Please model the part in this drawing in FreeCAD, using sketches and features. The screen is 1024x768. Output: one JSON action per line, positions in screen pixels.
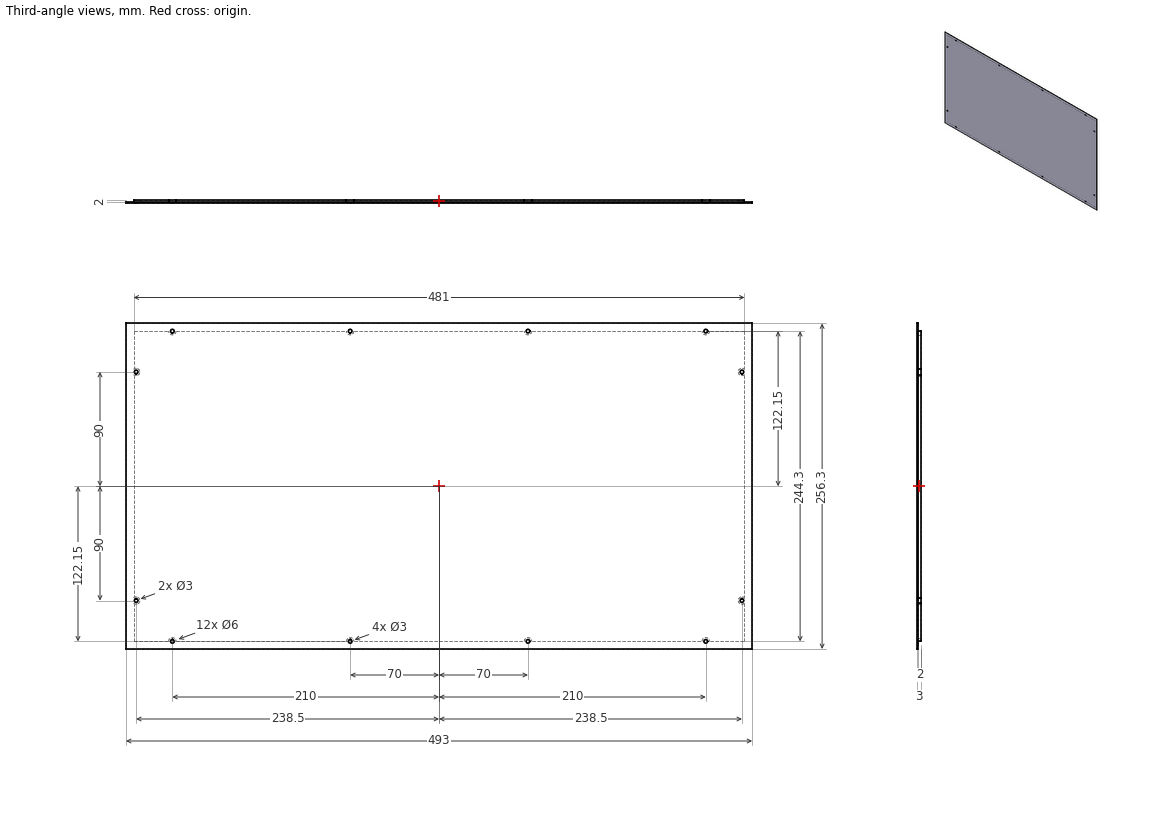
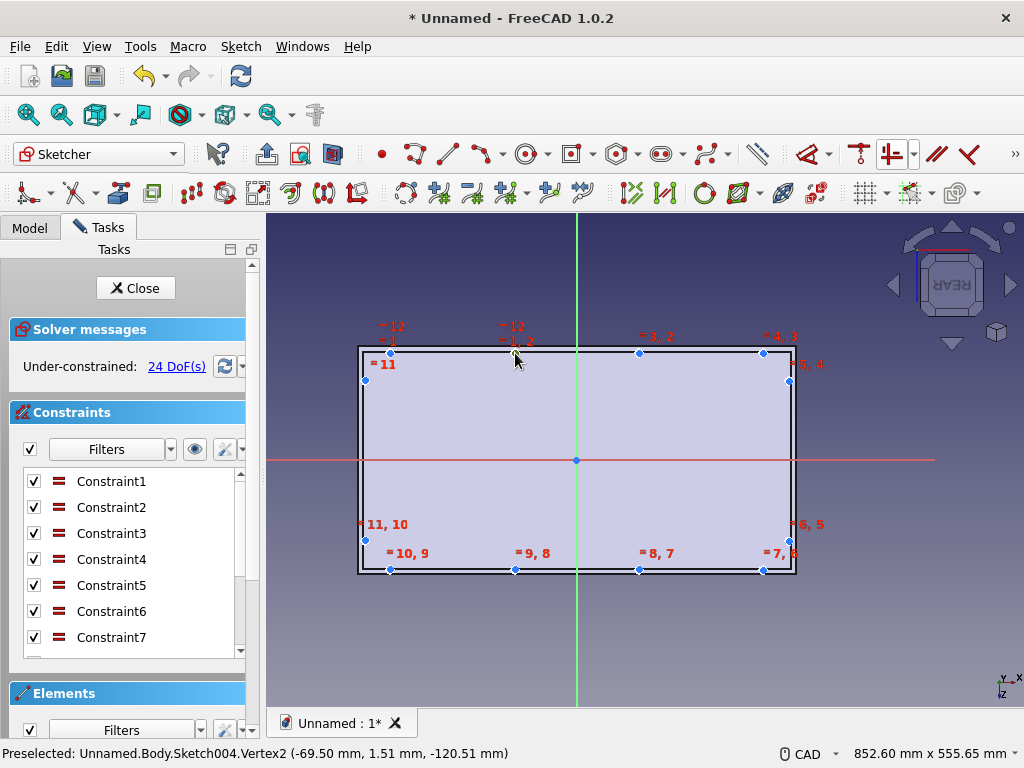
{"action": "left_click", "coordinate": [639, 353]}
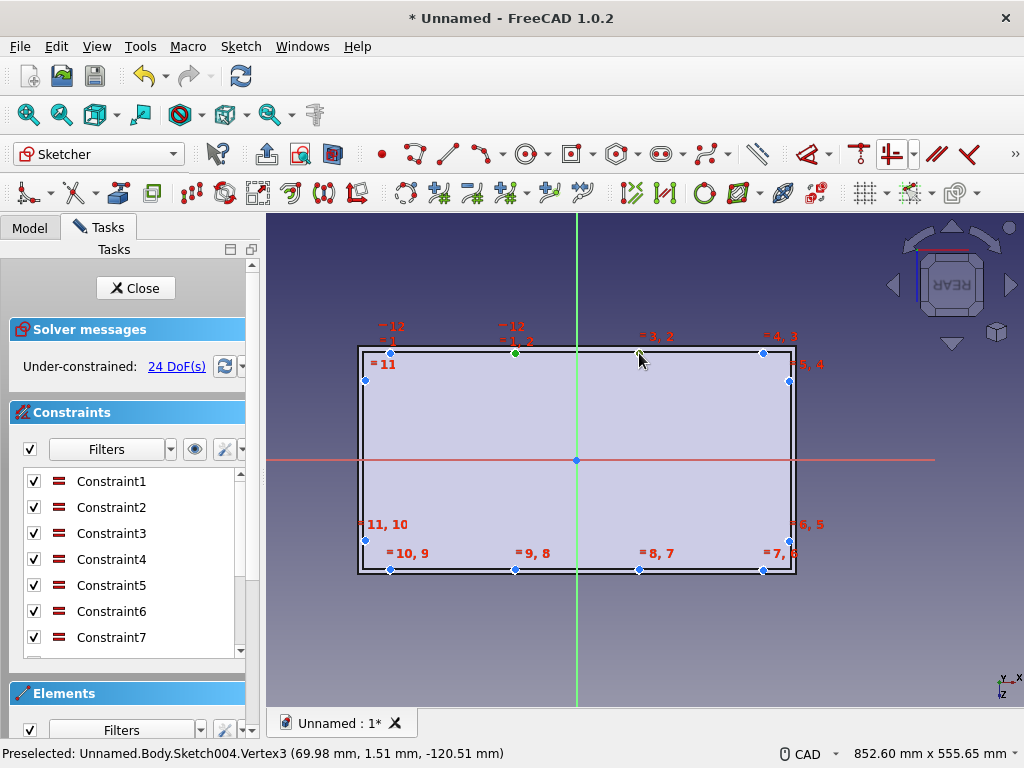
{"action": "left_click", "coordinate": [914, 154]}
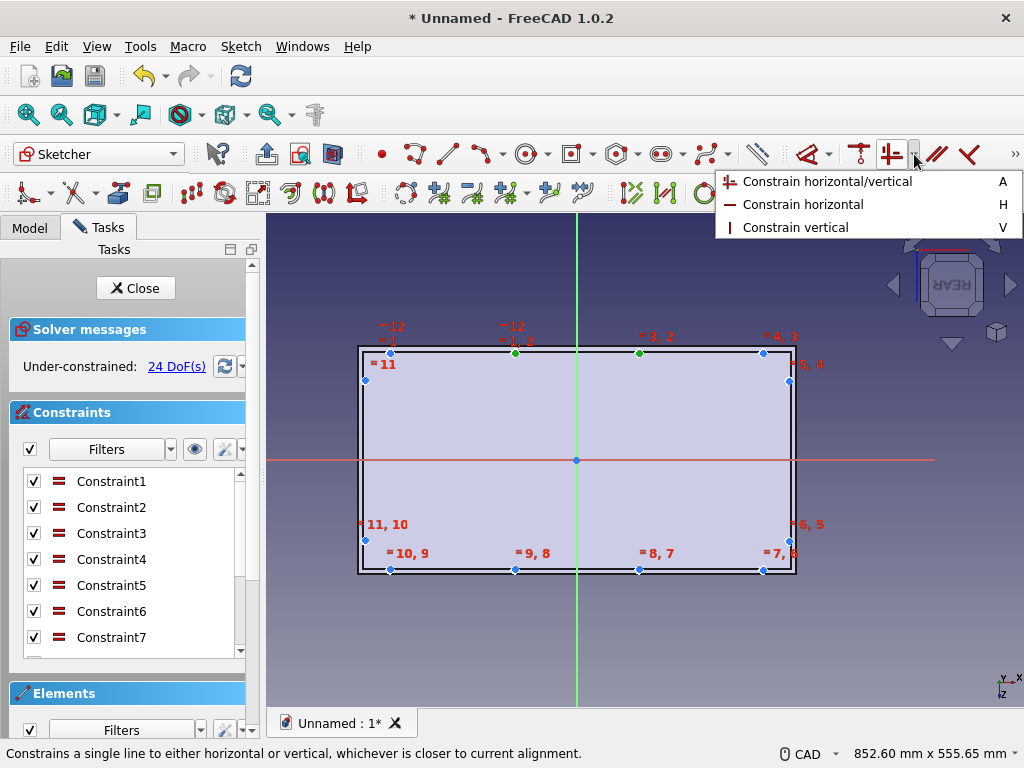
{"action": "left_click", "coordinate": [869, 204]}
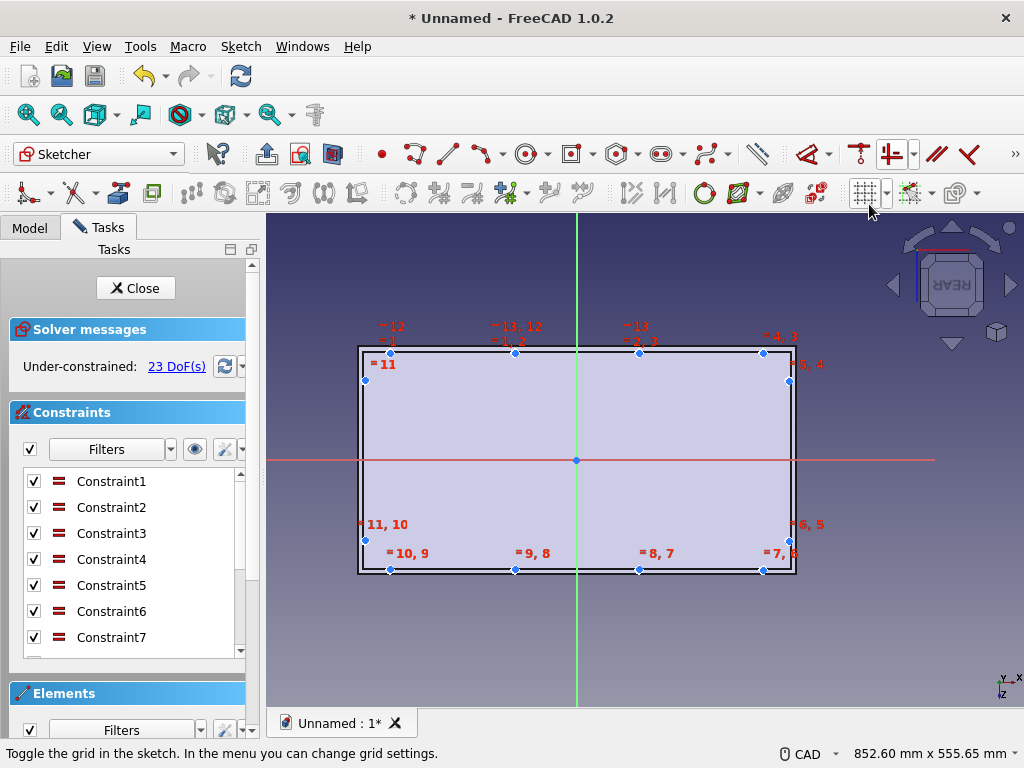
{"action": "left_click", "coordinate": [639, 353]}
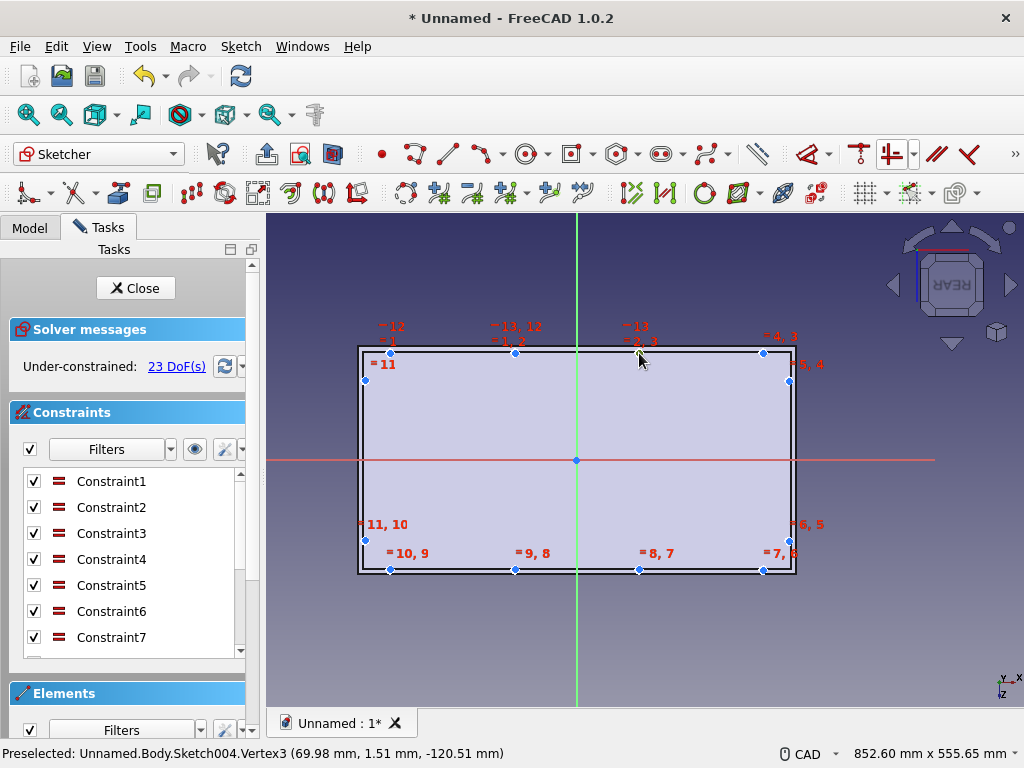
{"action": "left_click", "coordinate": [763, 353]}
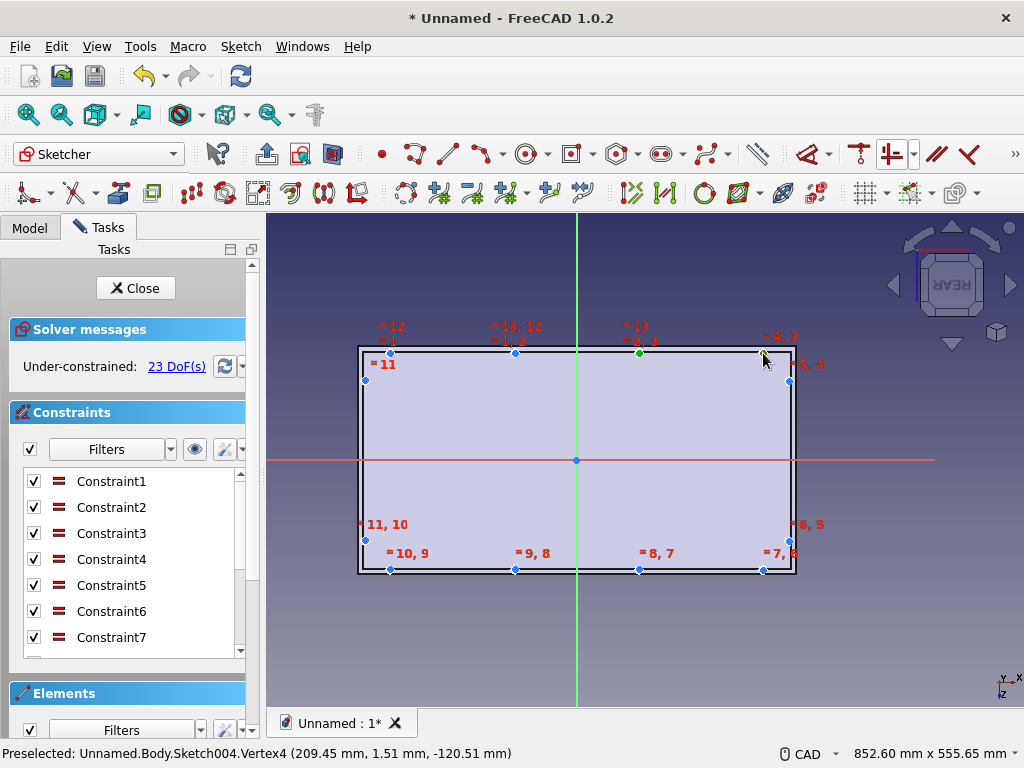
{"action": "left_click", "coordinate": [914, 154]}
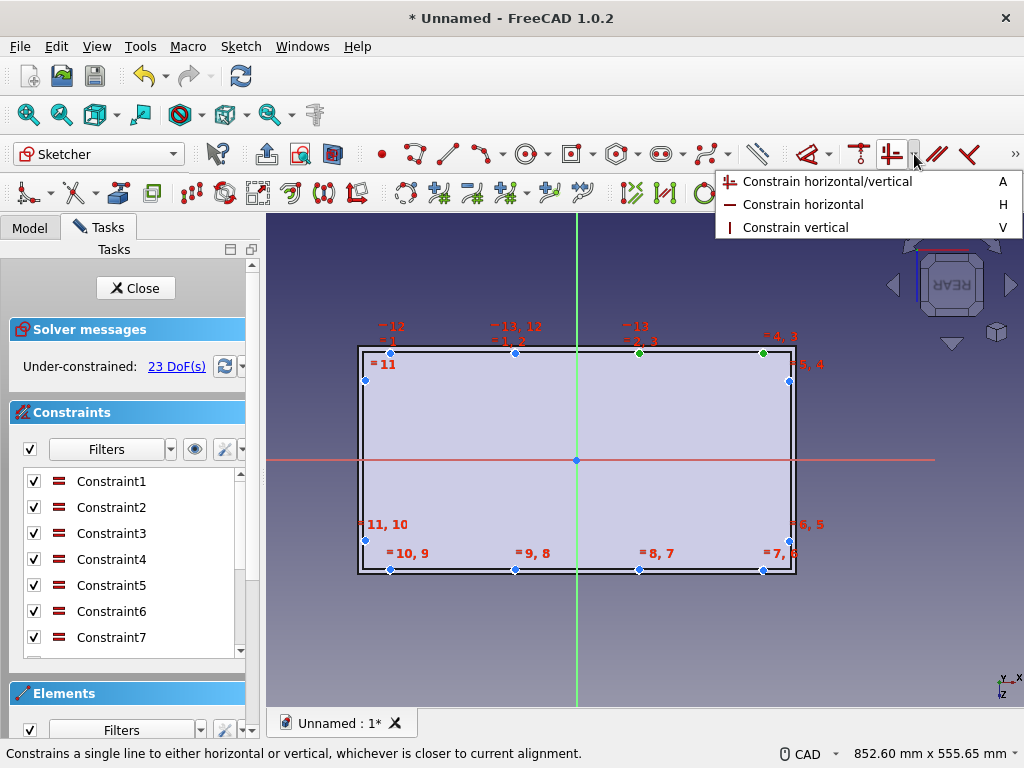
{"action": "left_click", "coordinate": [869, 204]}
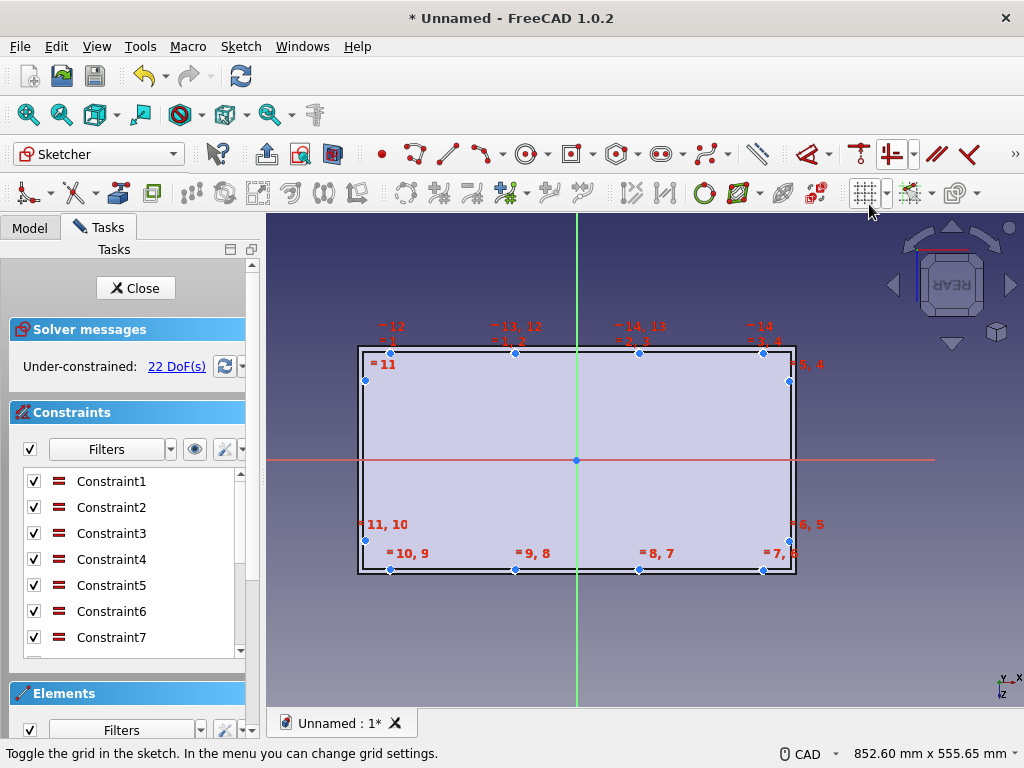
{"action": "left_click", "coordinate": [789, 381]}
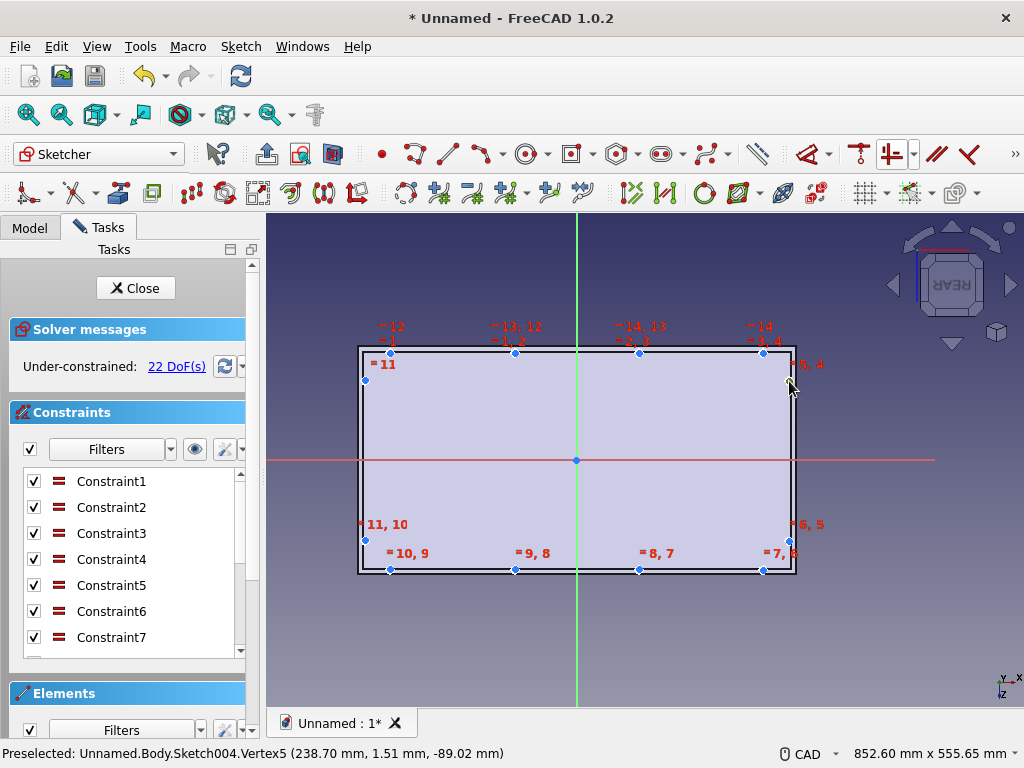
{"action": "left_click", "coordinate": [789, 541]}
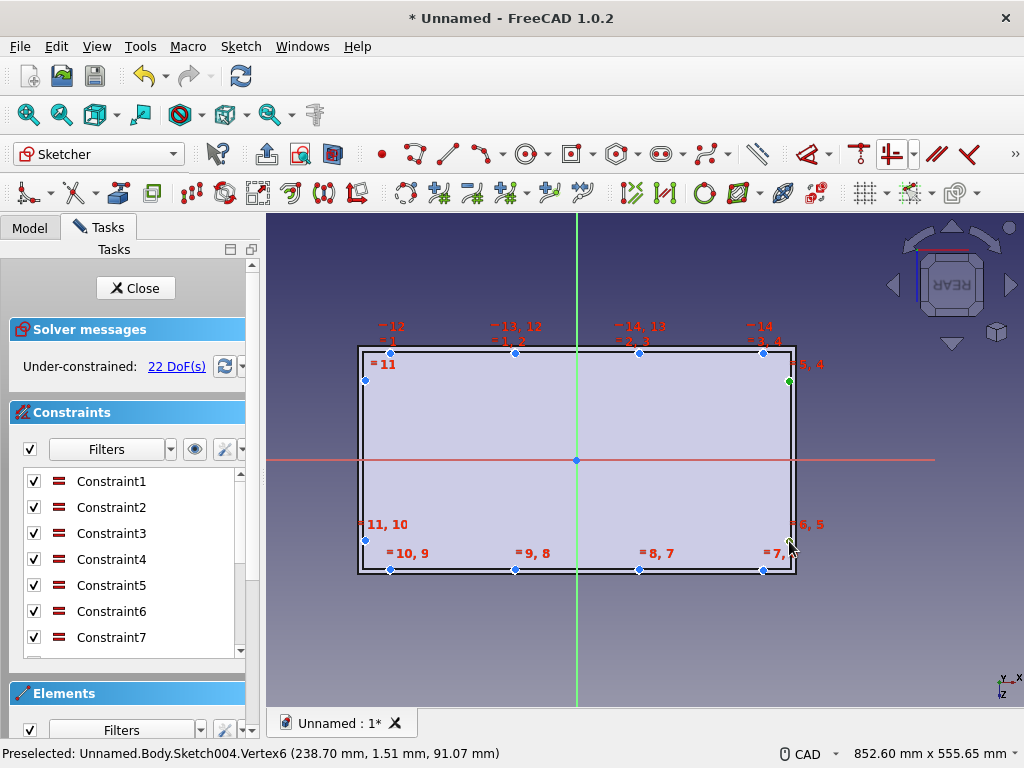
{"action": "key", "text": "v"}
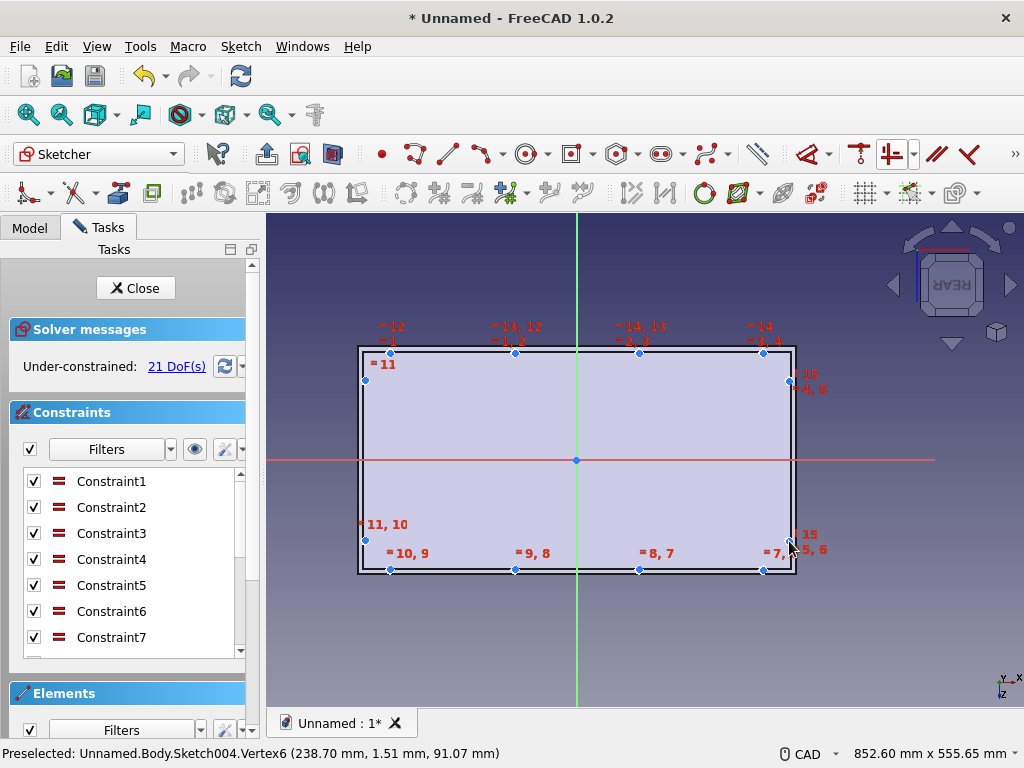
{"action": "left_click", "coordinate": [763, 353]}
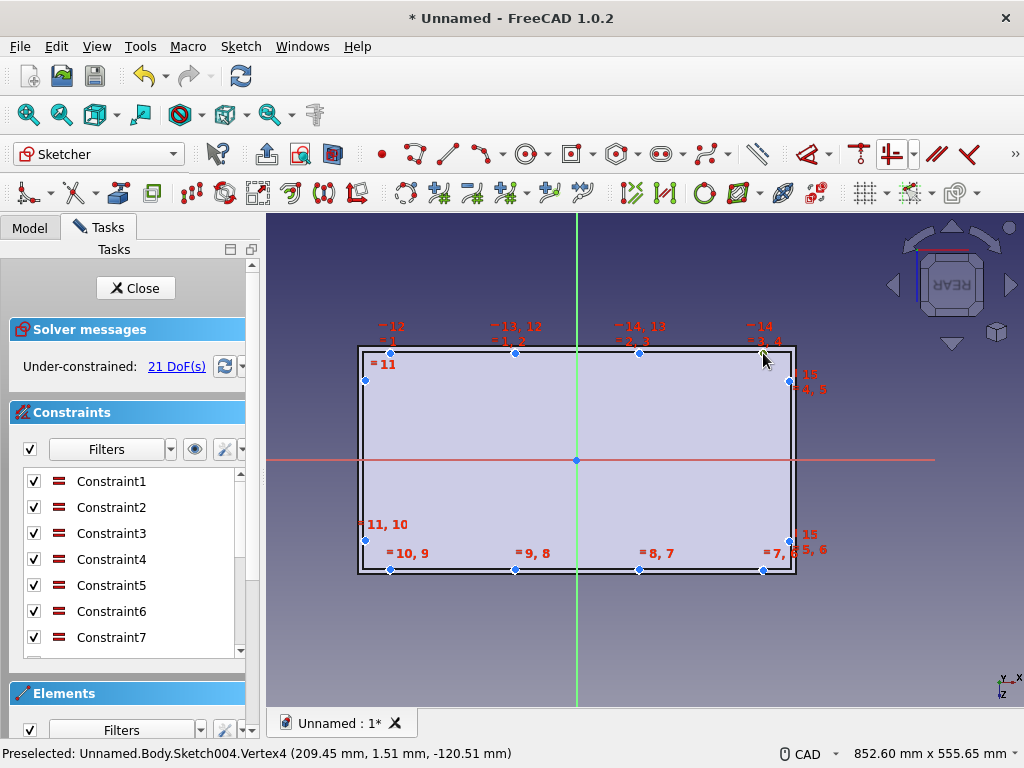
{"action": "left_click", "coordinate": [763, 570]}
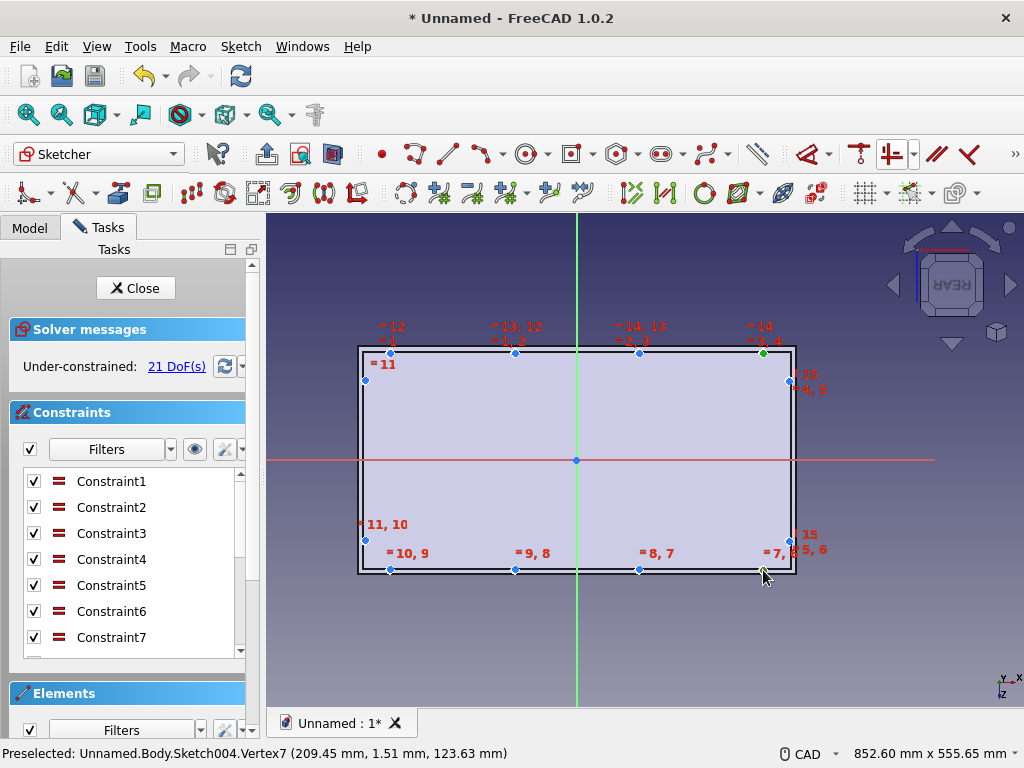
{"action": "key", "text": "v"}